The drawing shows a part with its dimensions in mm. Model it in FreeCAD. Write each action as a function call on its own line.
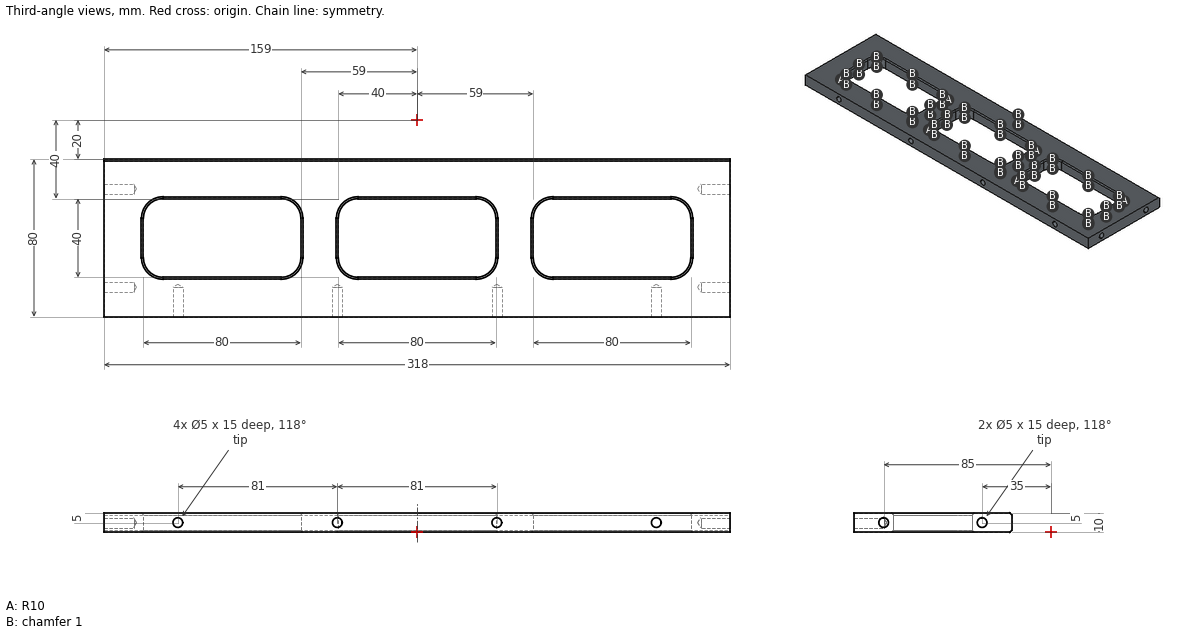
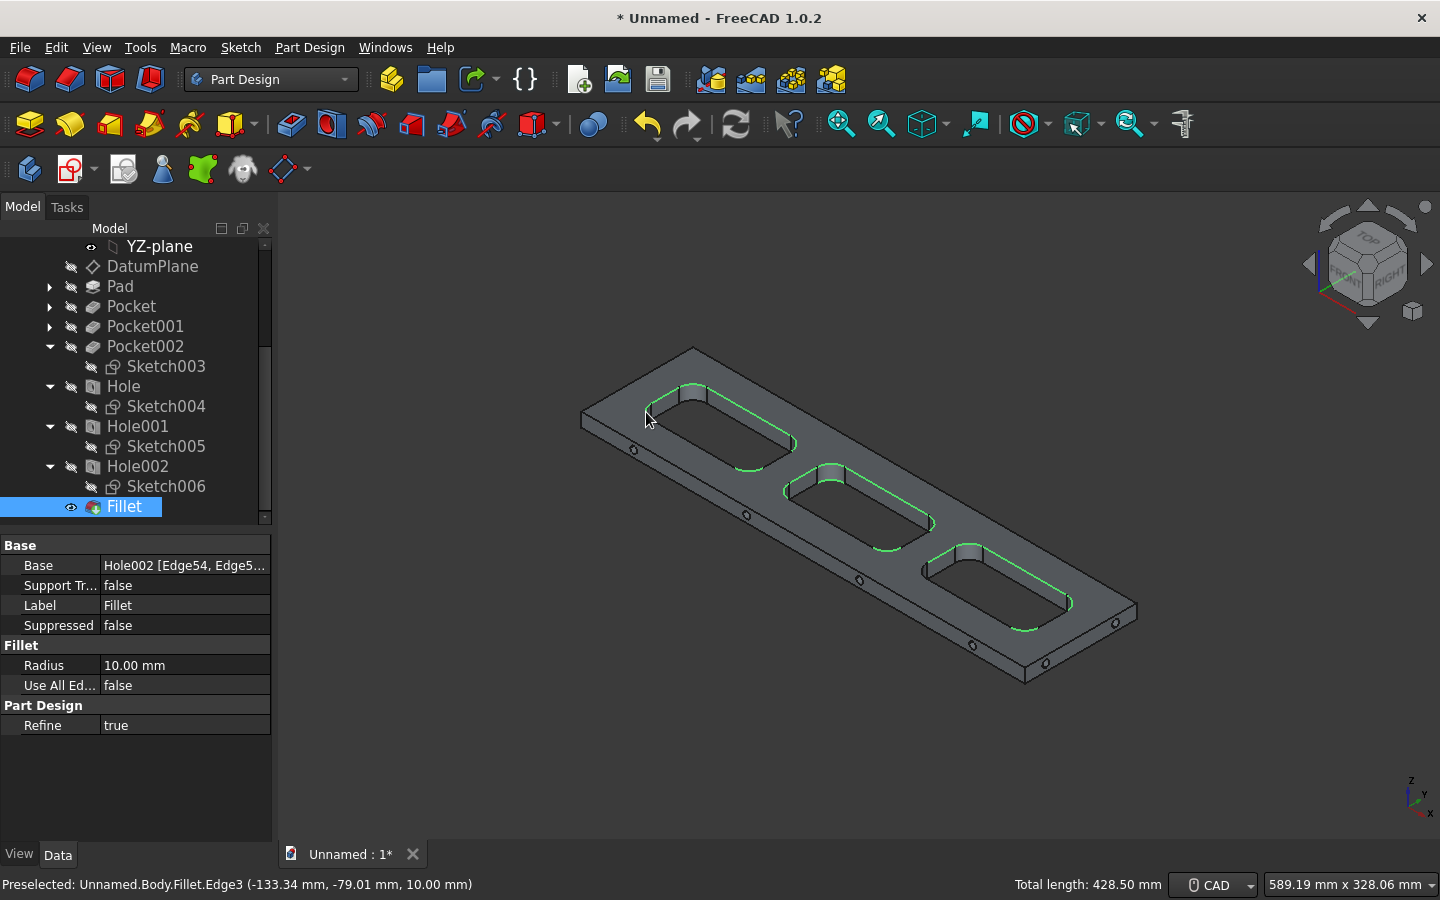
click(922, 570, ctrl)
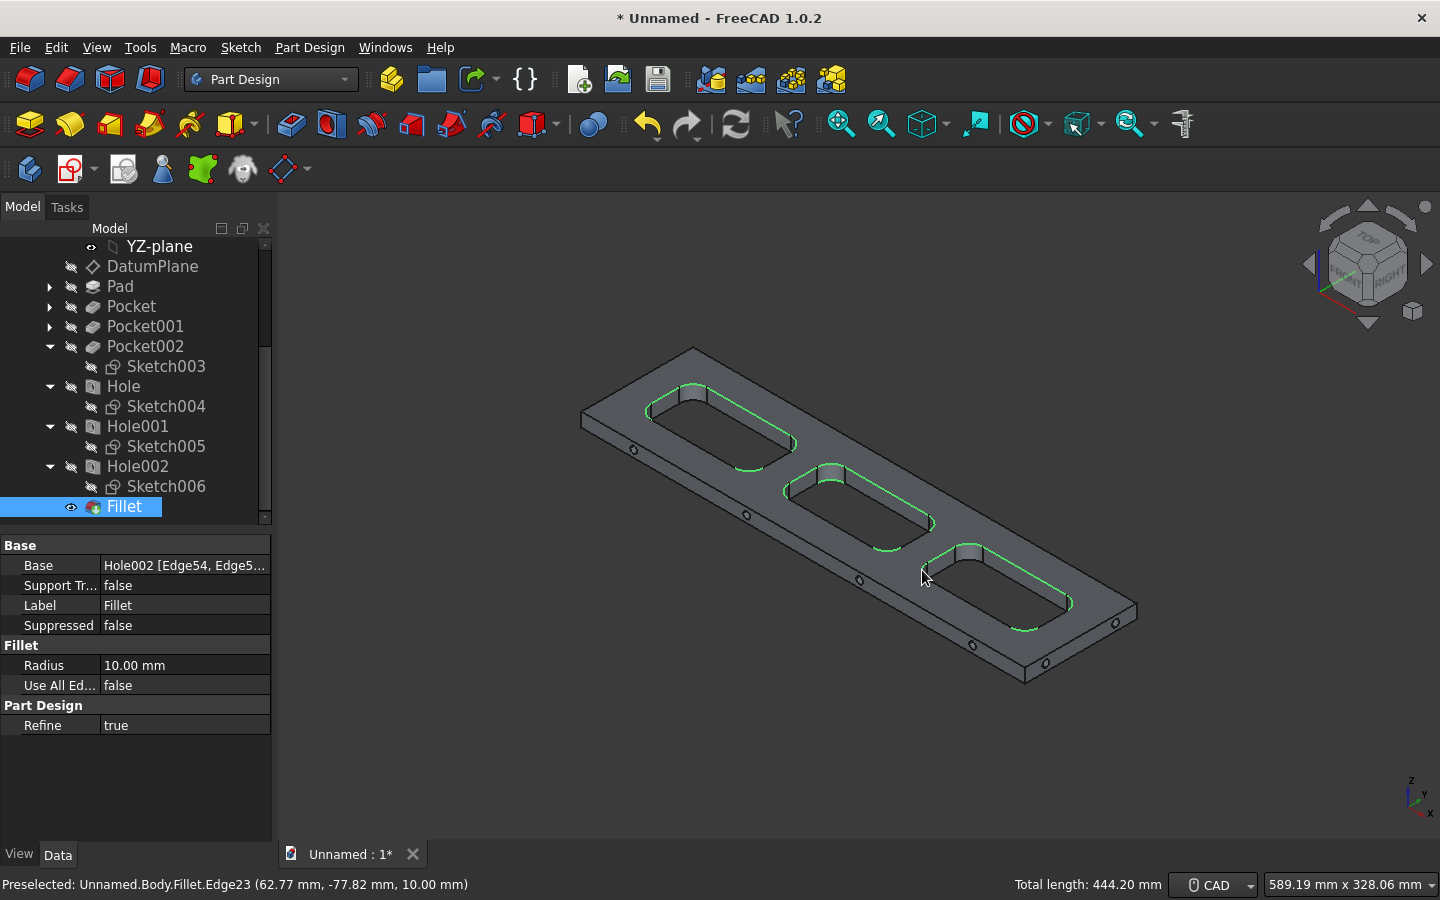
key(2)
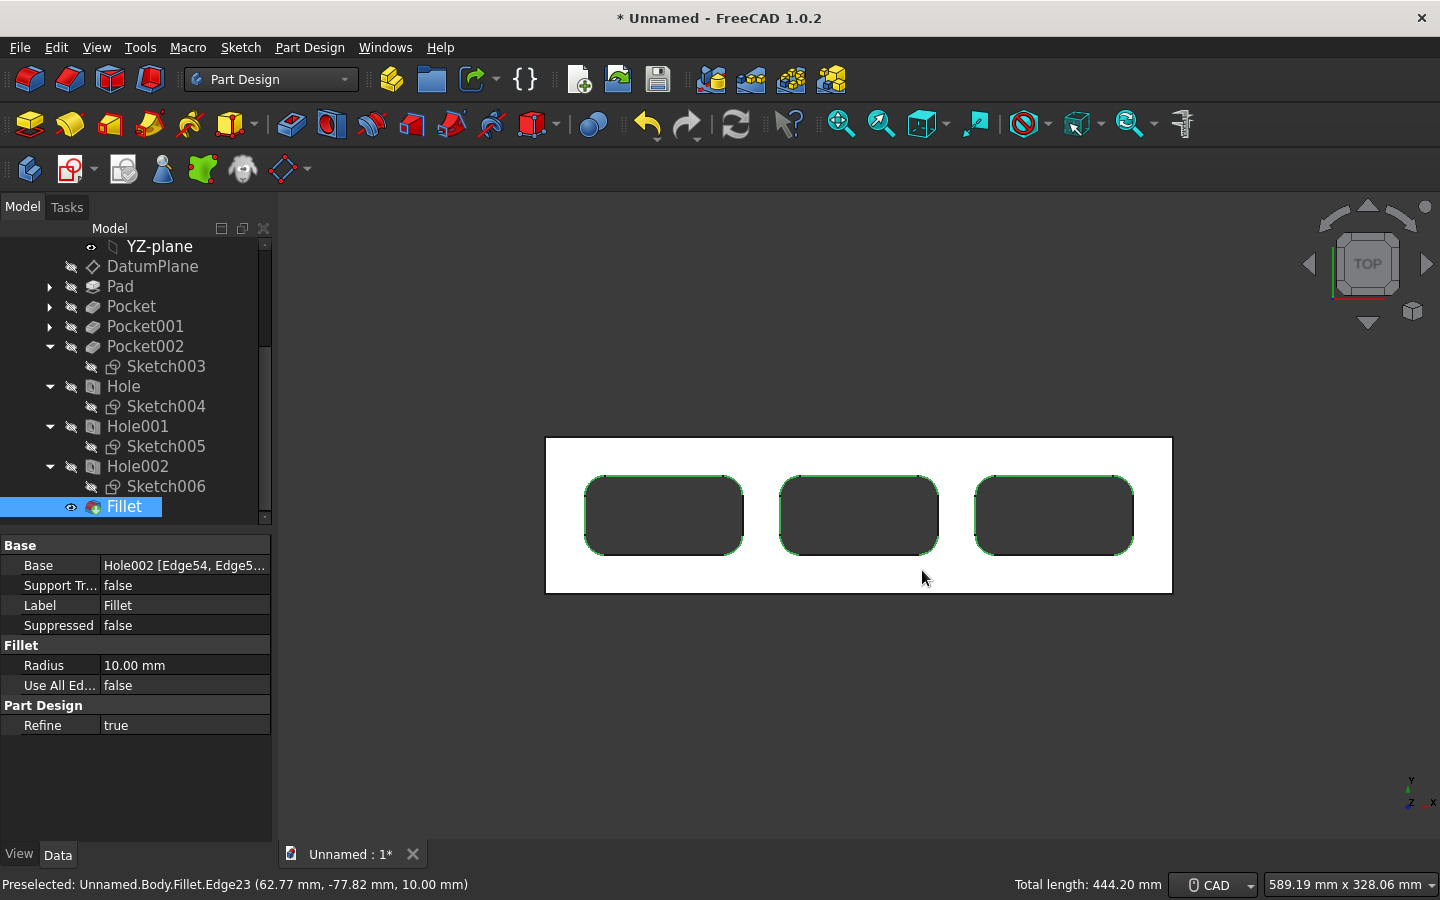
click(938, 514, ctrl)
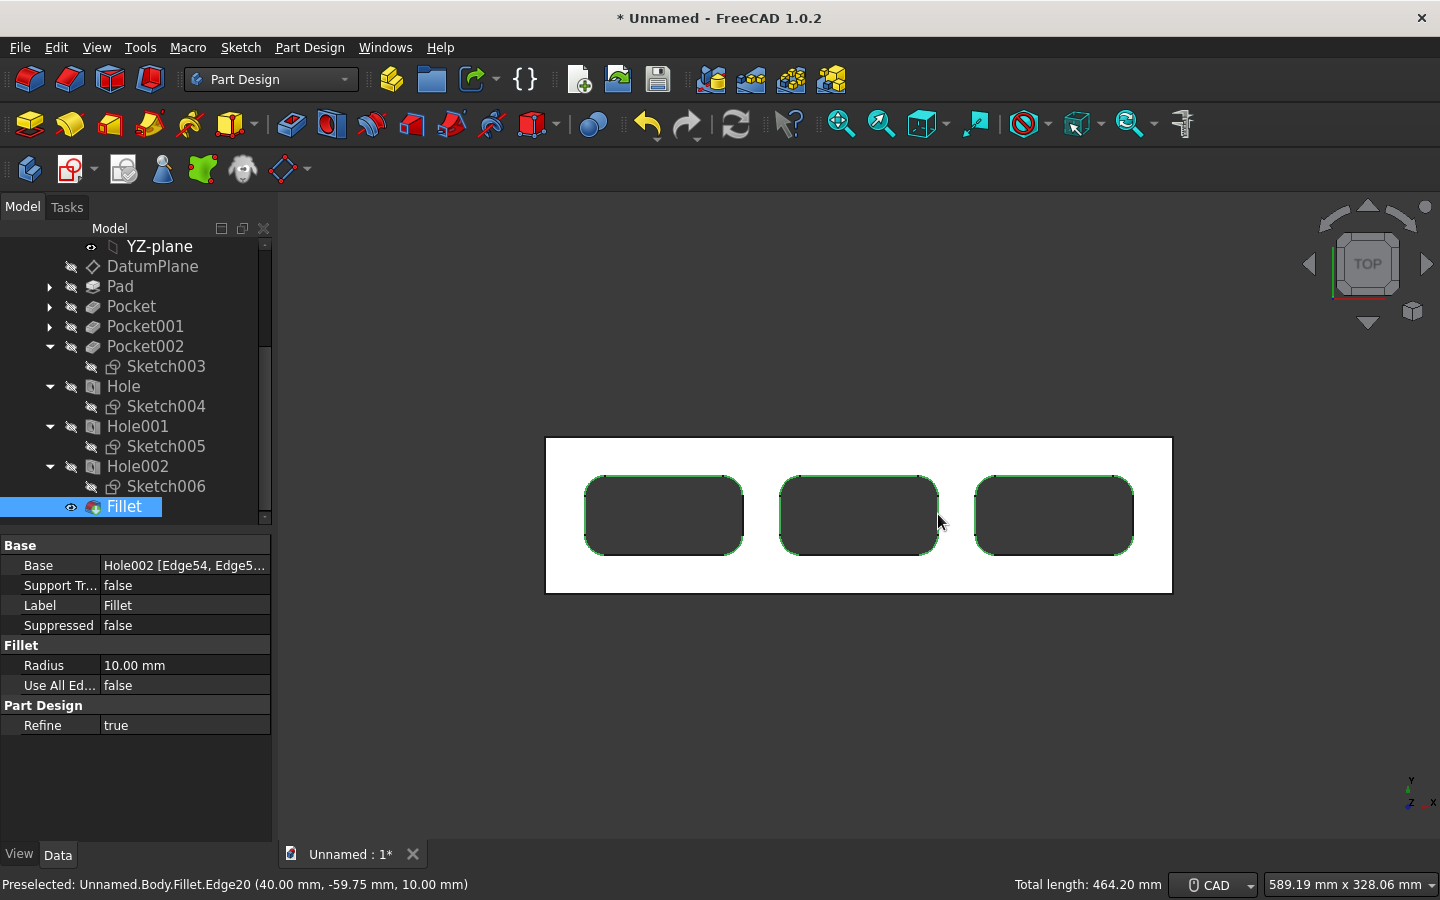
click(1133, 514, ctrl)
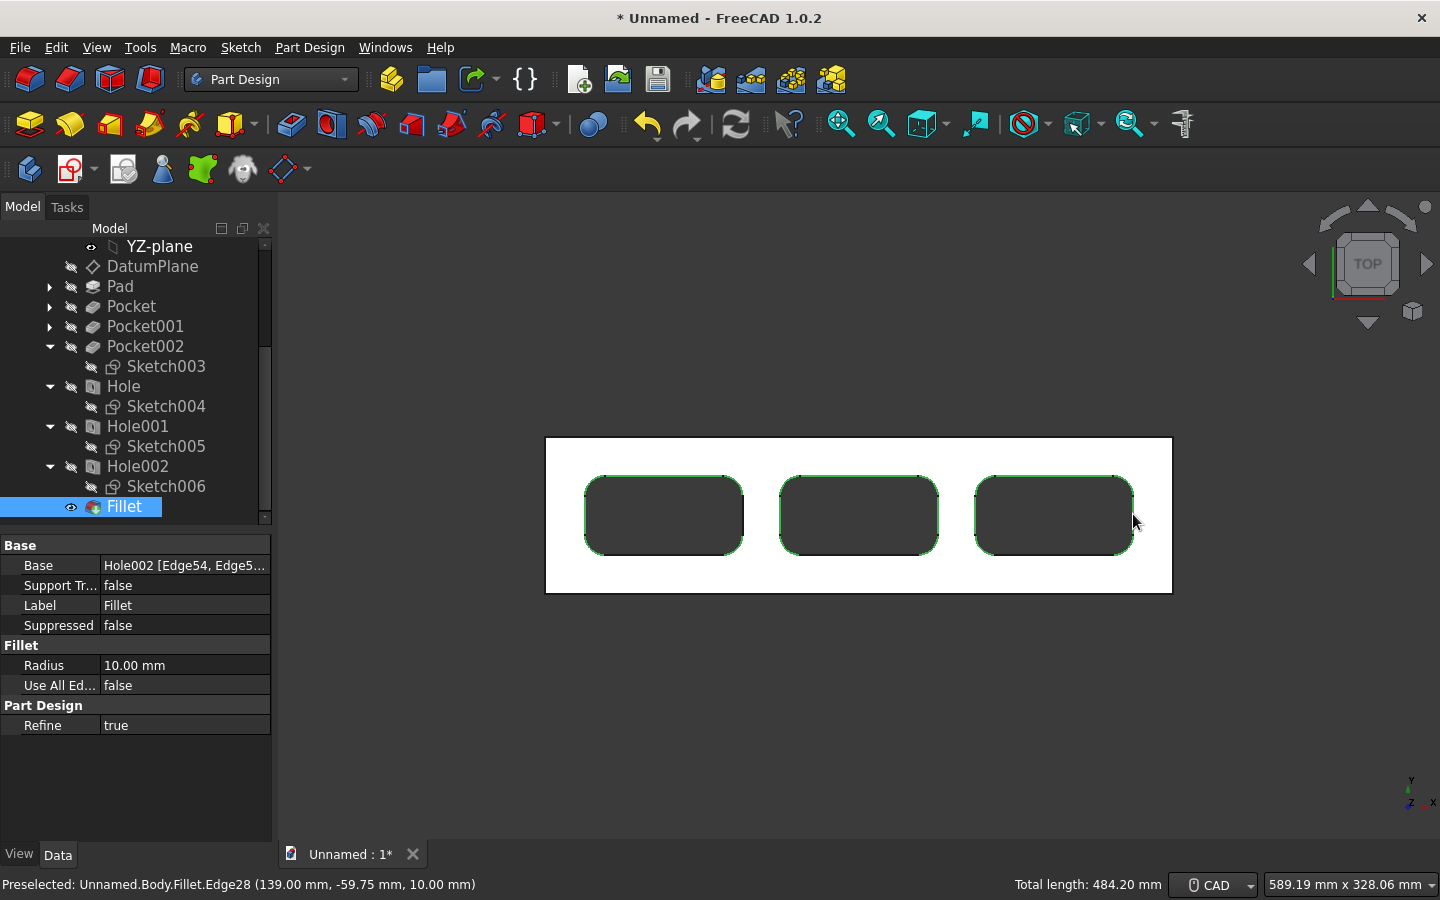
click(859, 554, ctrl)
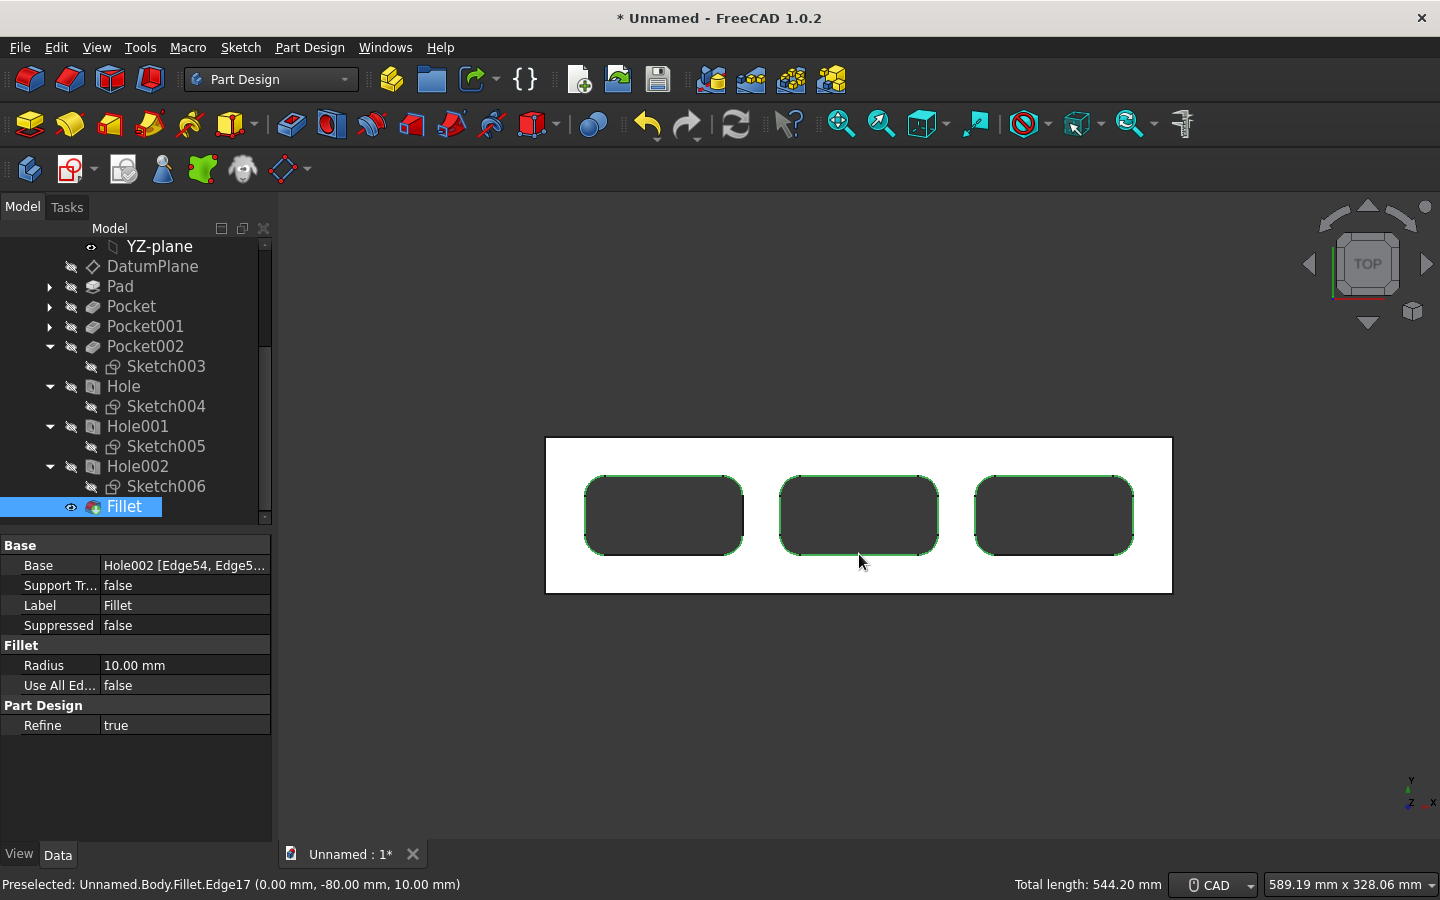
click(1054, 554, ctrl)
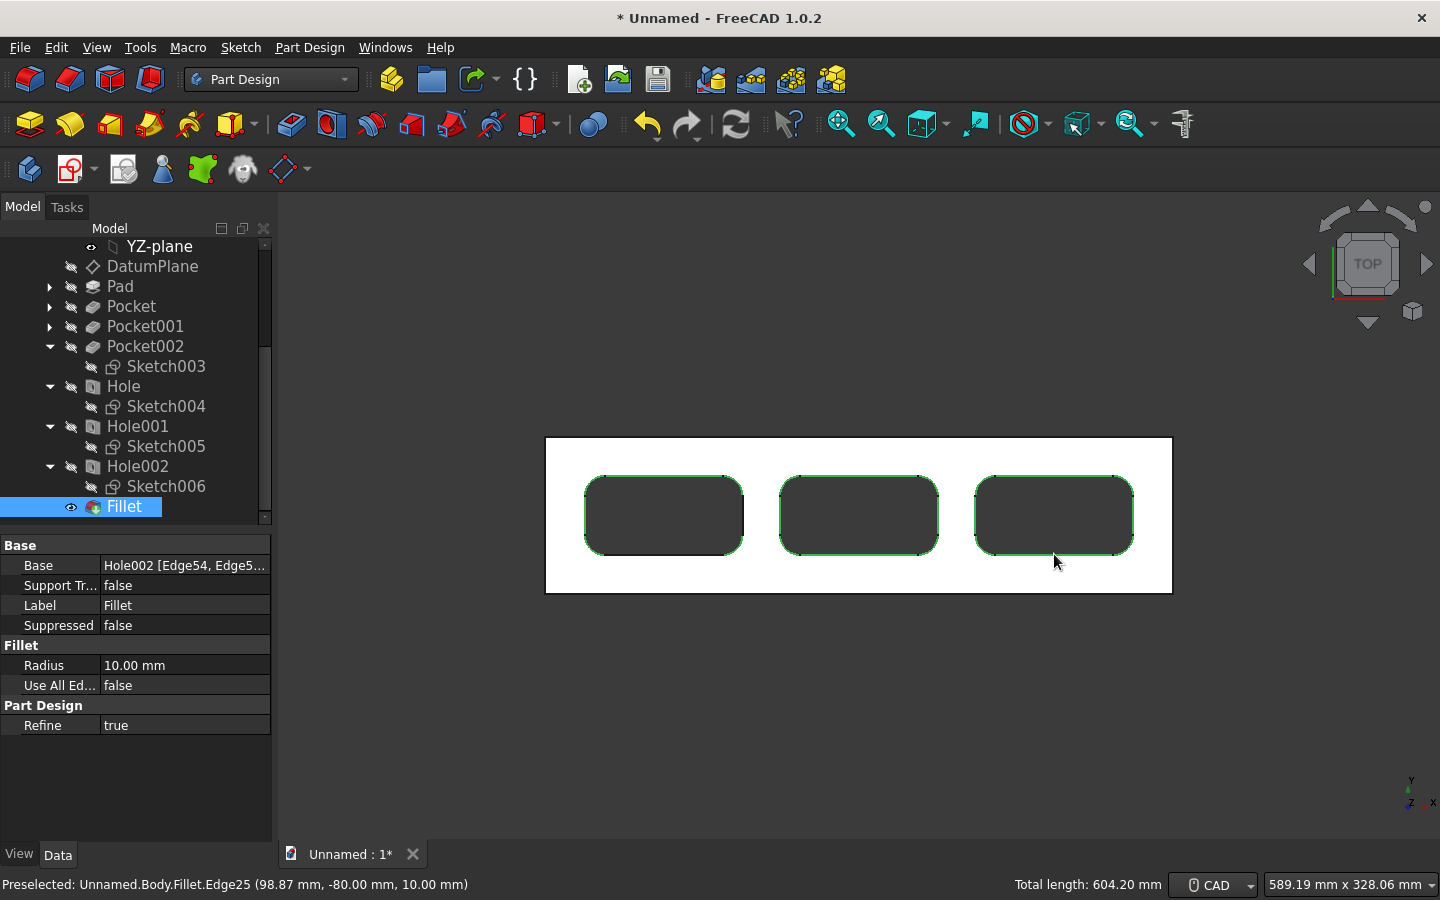
click(743, 514, ctrl)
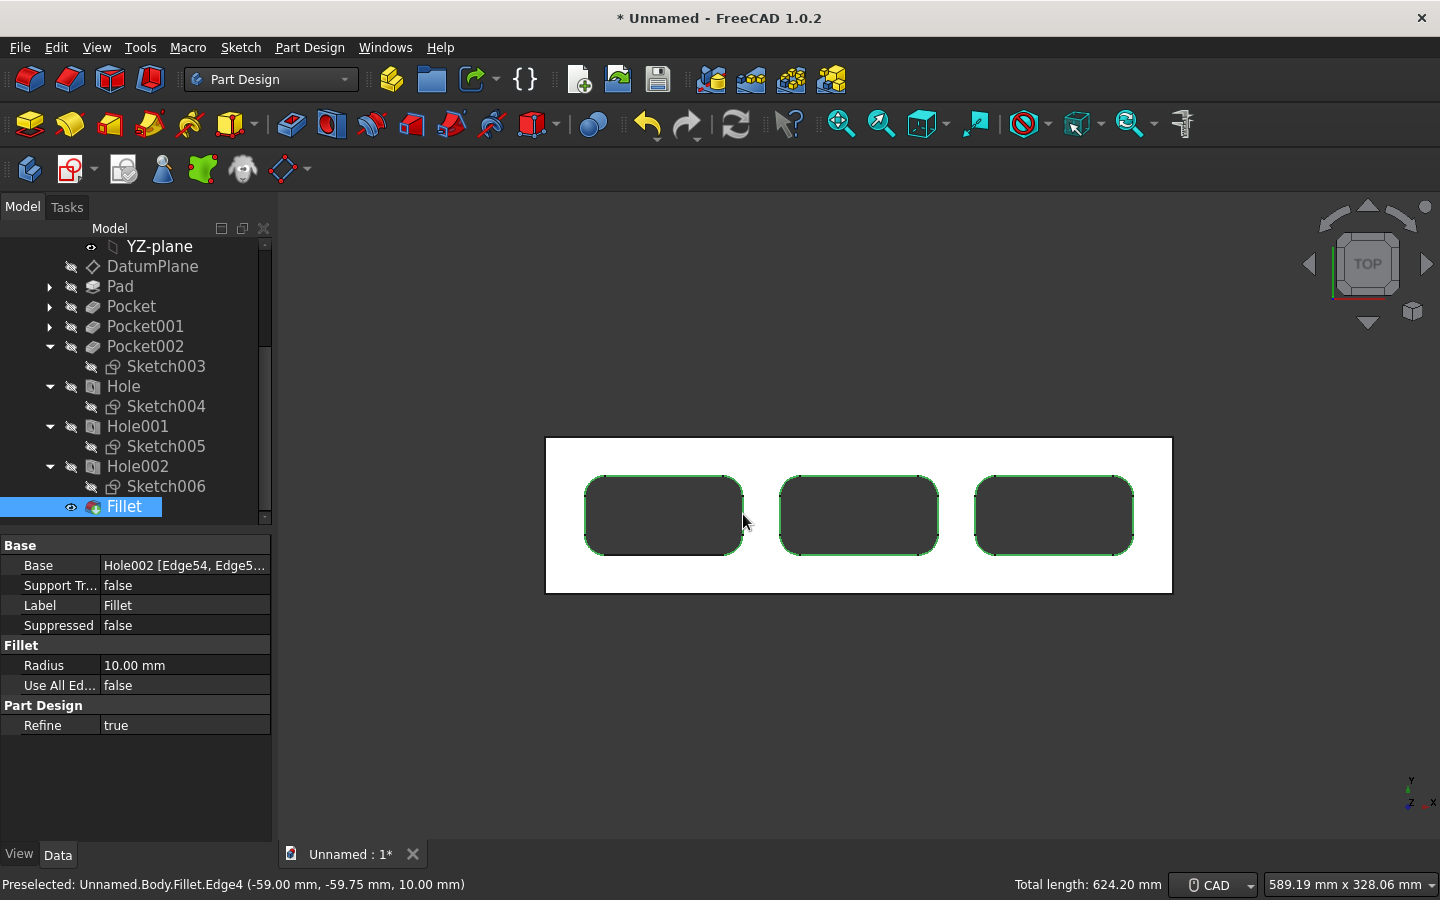
click(664, 554, ctrl)